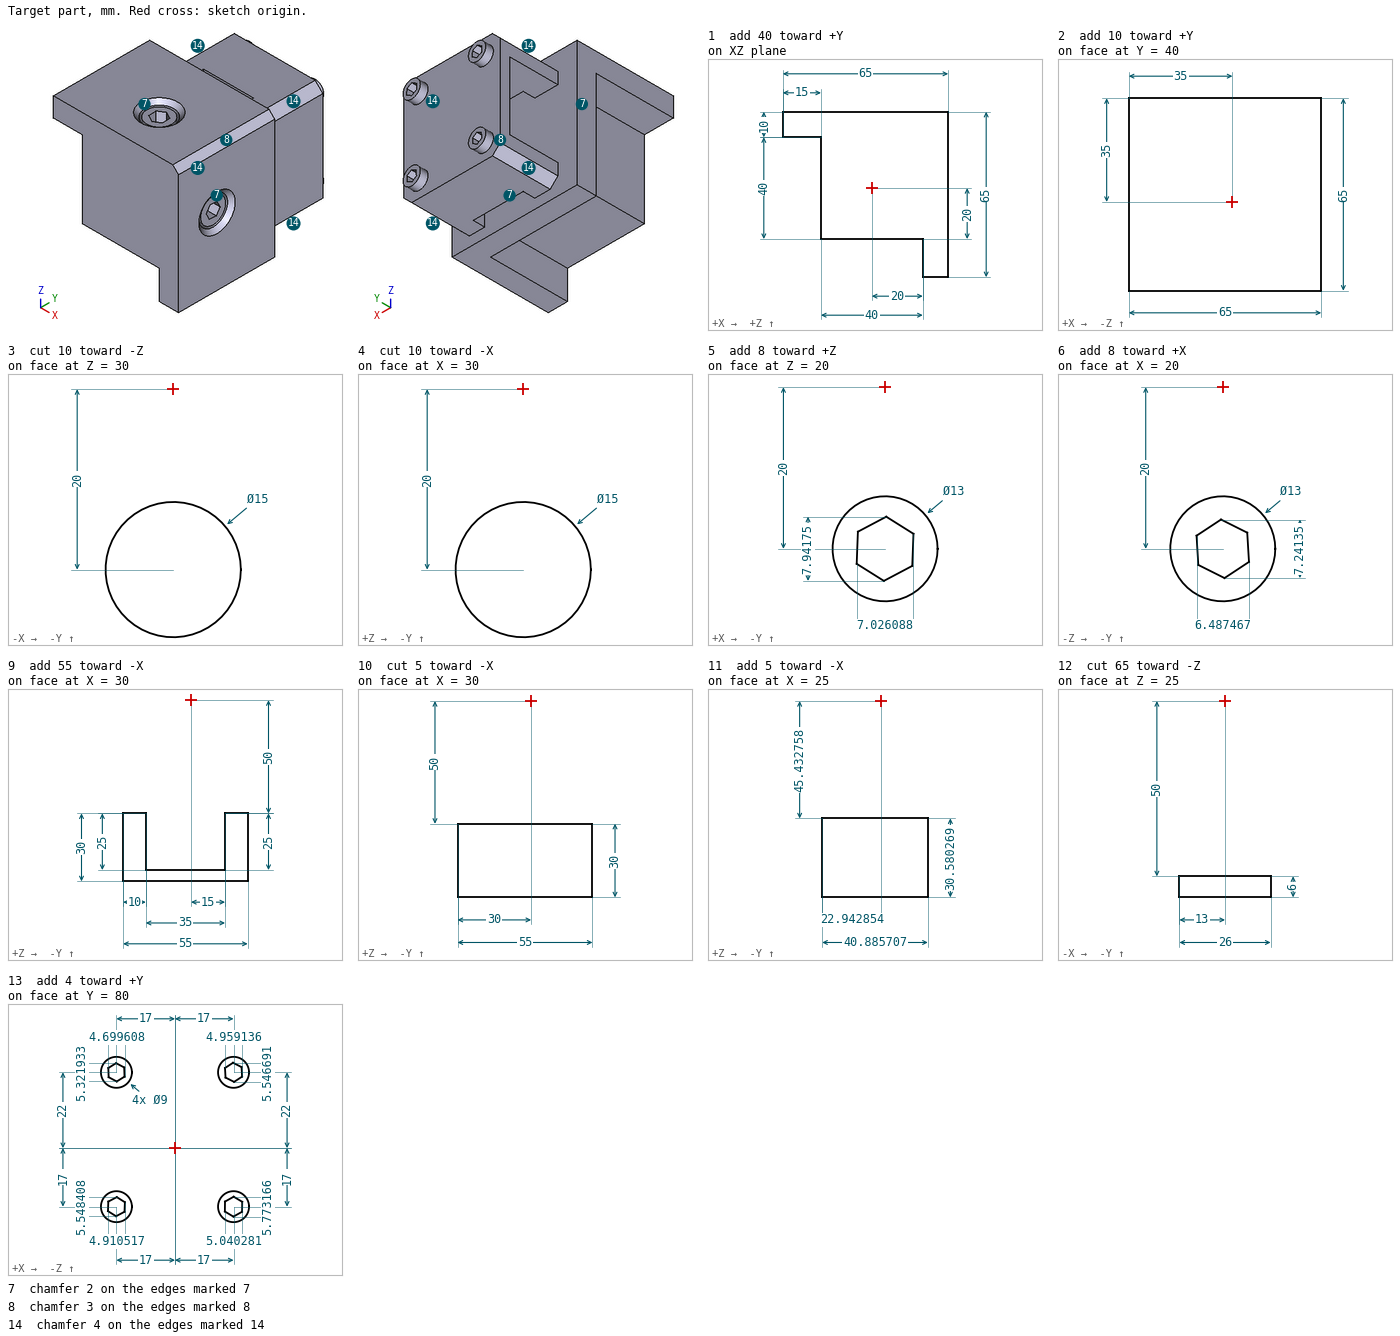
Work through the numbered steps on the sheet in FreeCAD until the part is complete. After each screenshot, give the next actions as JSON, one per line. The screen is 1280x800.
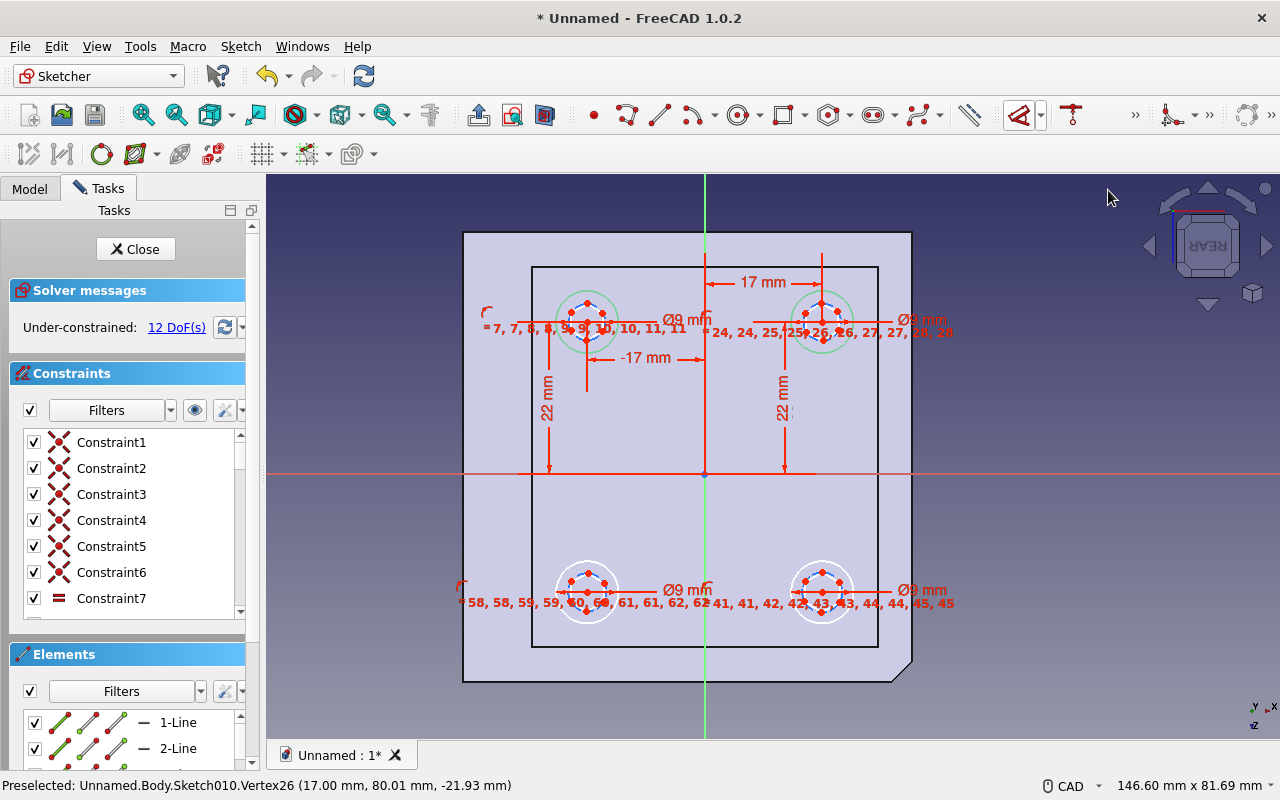
{"action": "left_click", "coordinate": [822, 592]}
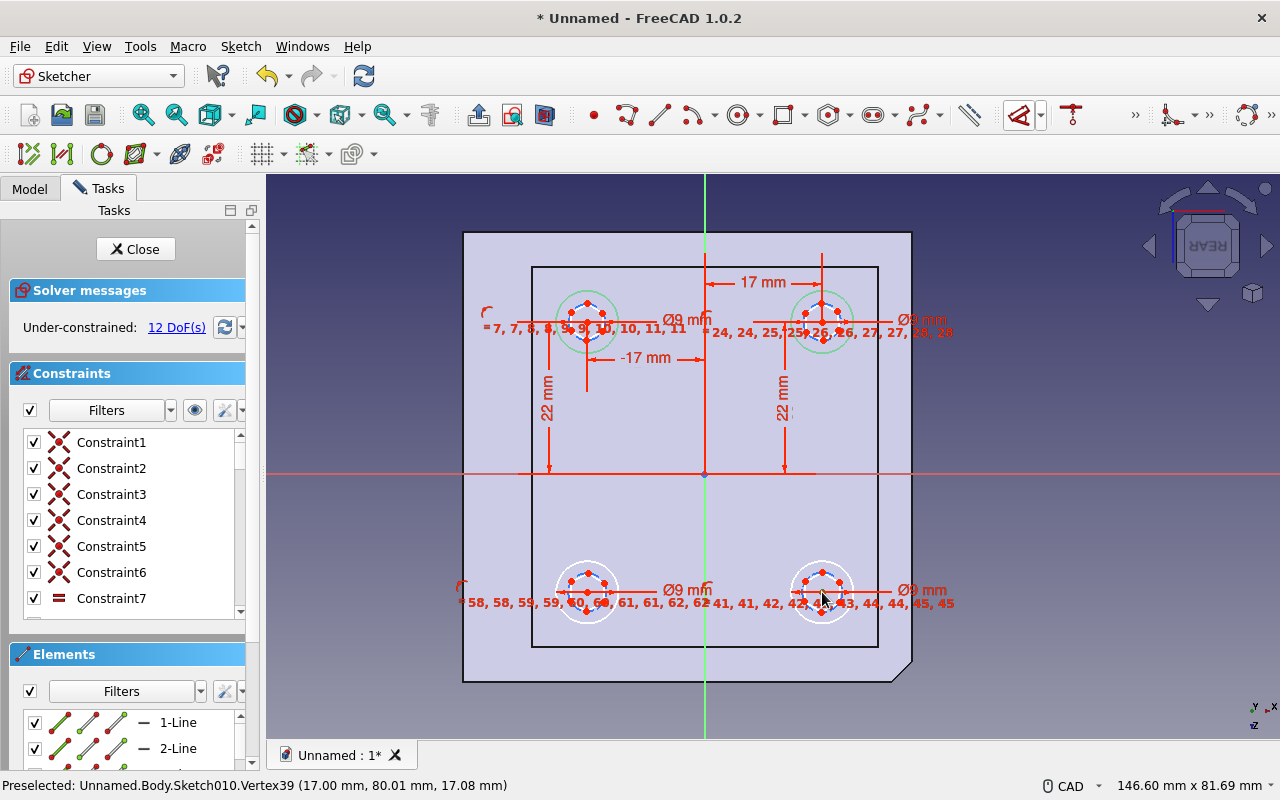
{"action": "left_click", "coordinate": [1040, 116]}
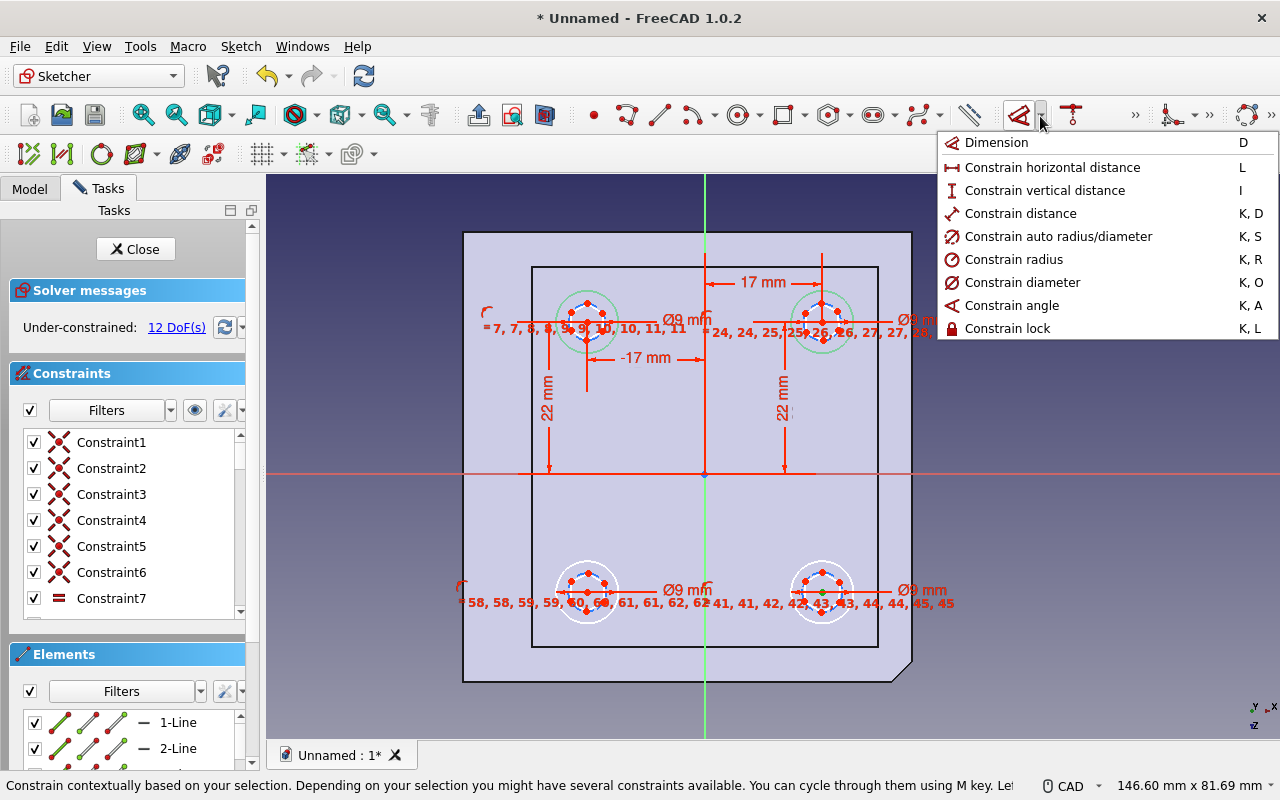
{"action": "left_click", "coordinate": [1108, 168]}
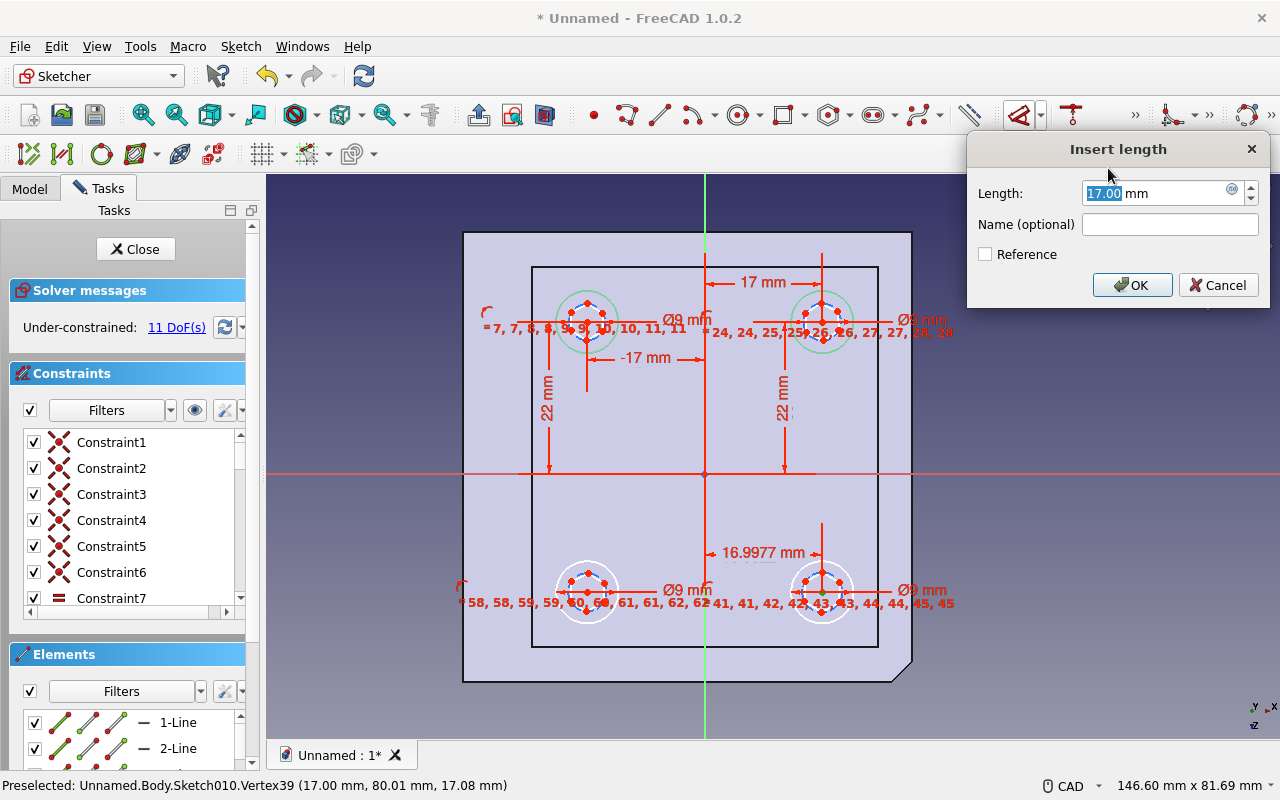
{"action": "type", "text": "17"}
{"action": "key", "text": "Return"}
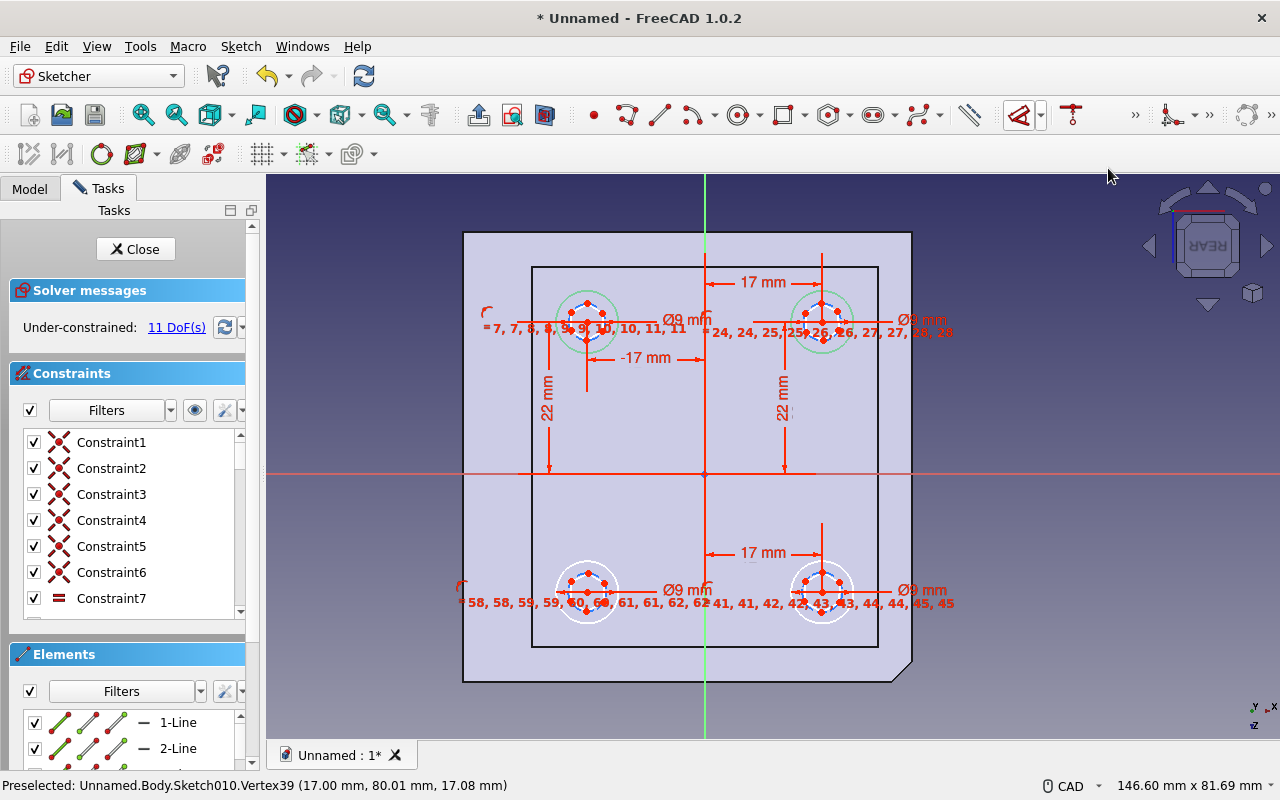
{"action": "left_click", "coordinate": [822, 592]}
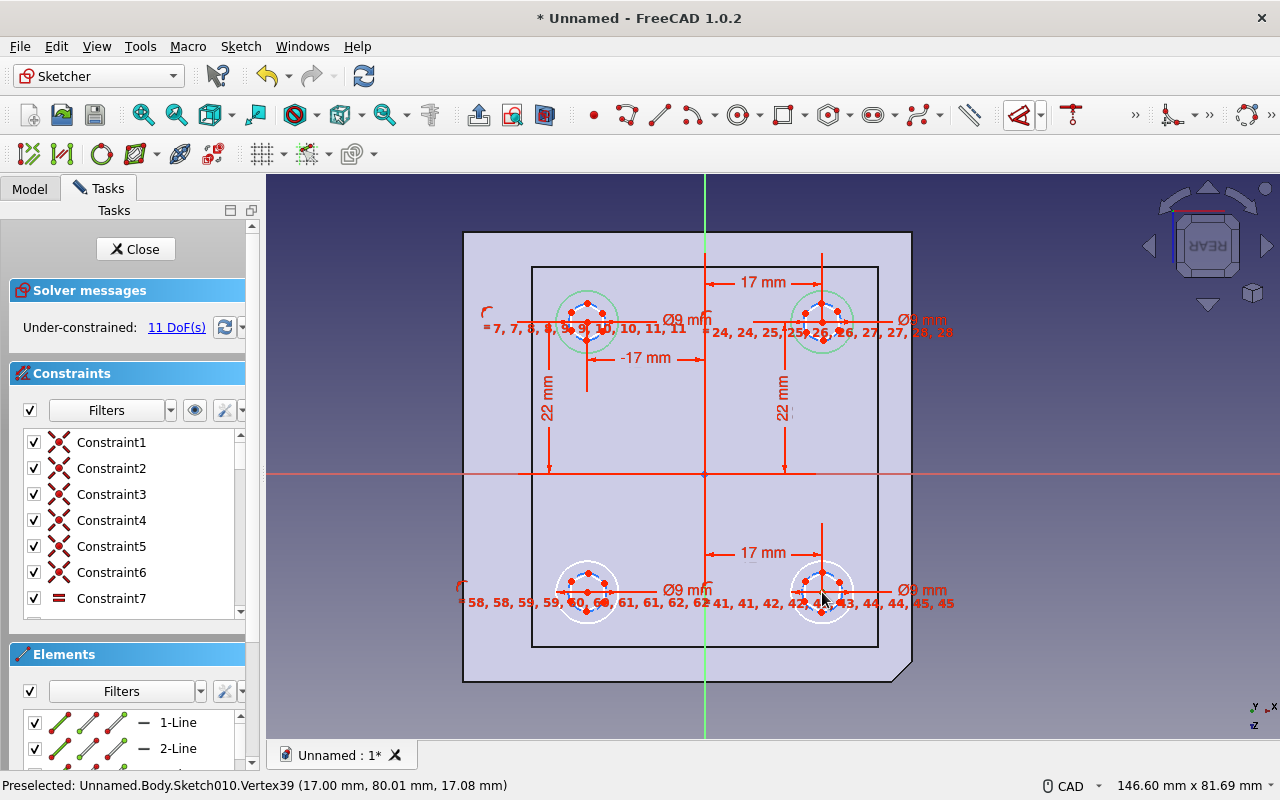
{"action": "key", "text": "i"}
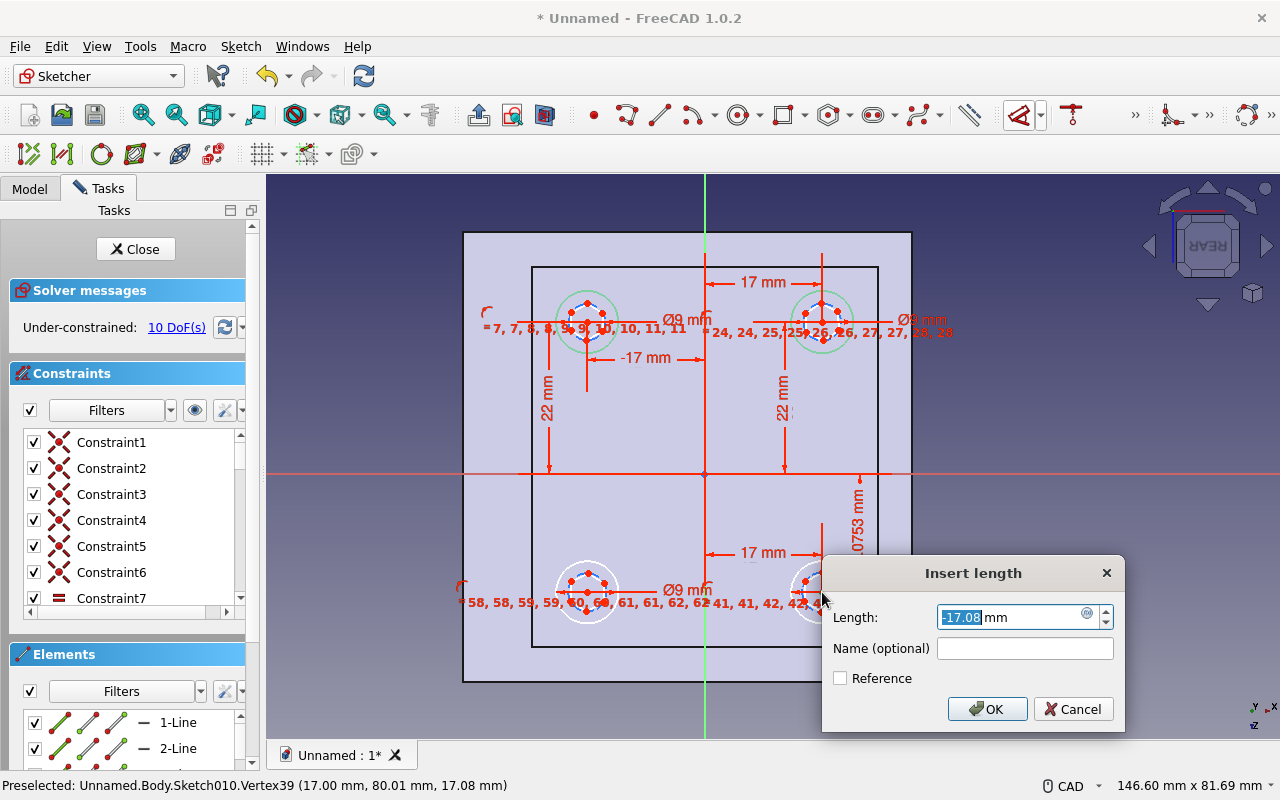
{"action": "type", "text": "-17"}
{"action": "key", "text": "Return"}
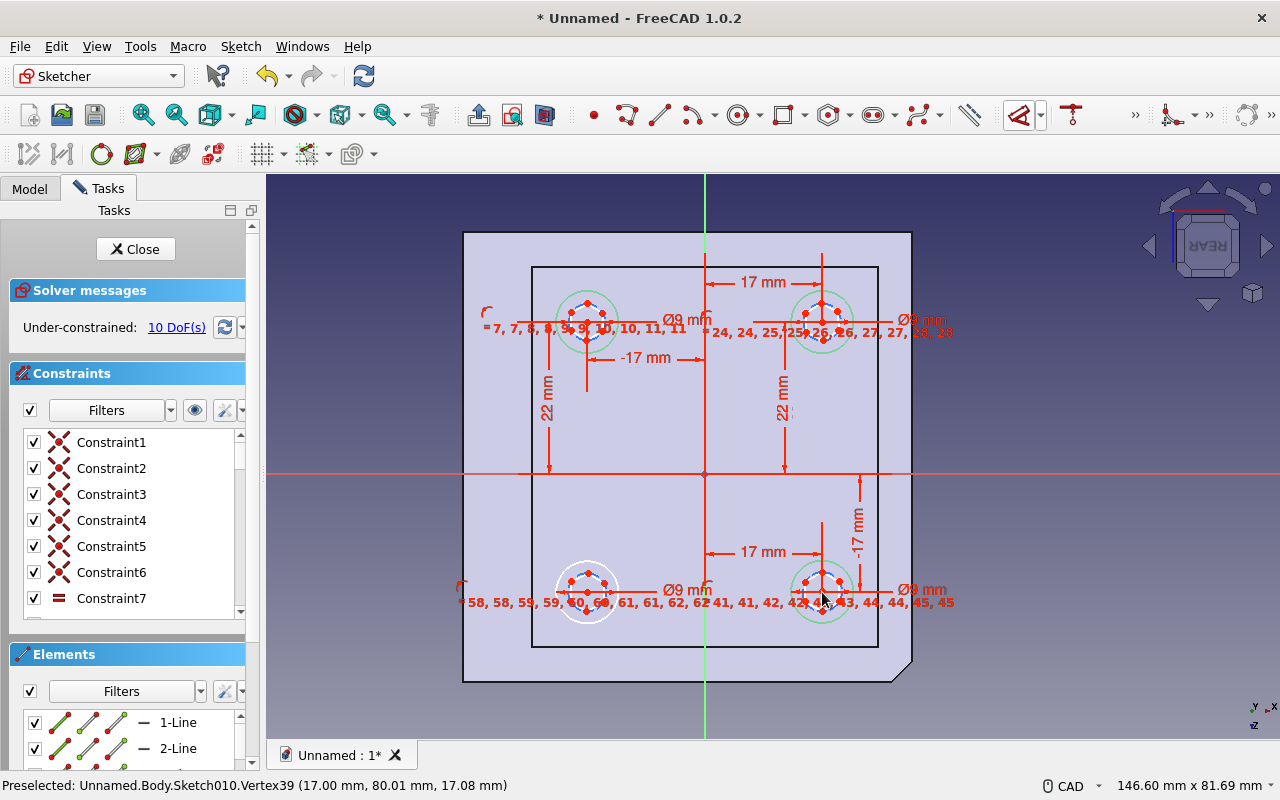
{"action": "left_click", "coordinate": [587, 592]}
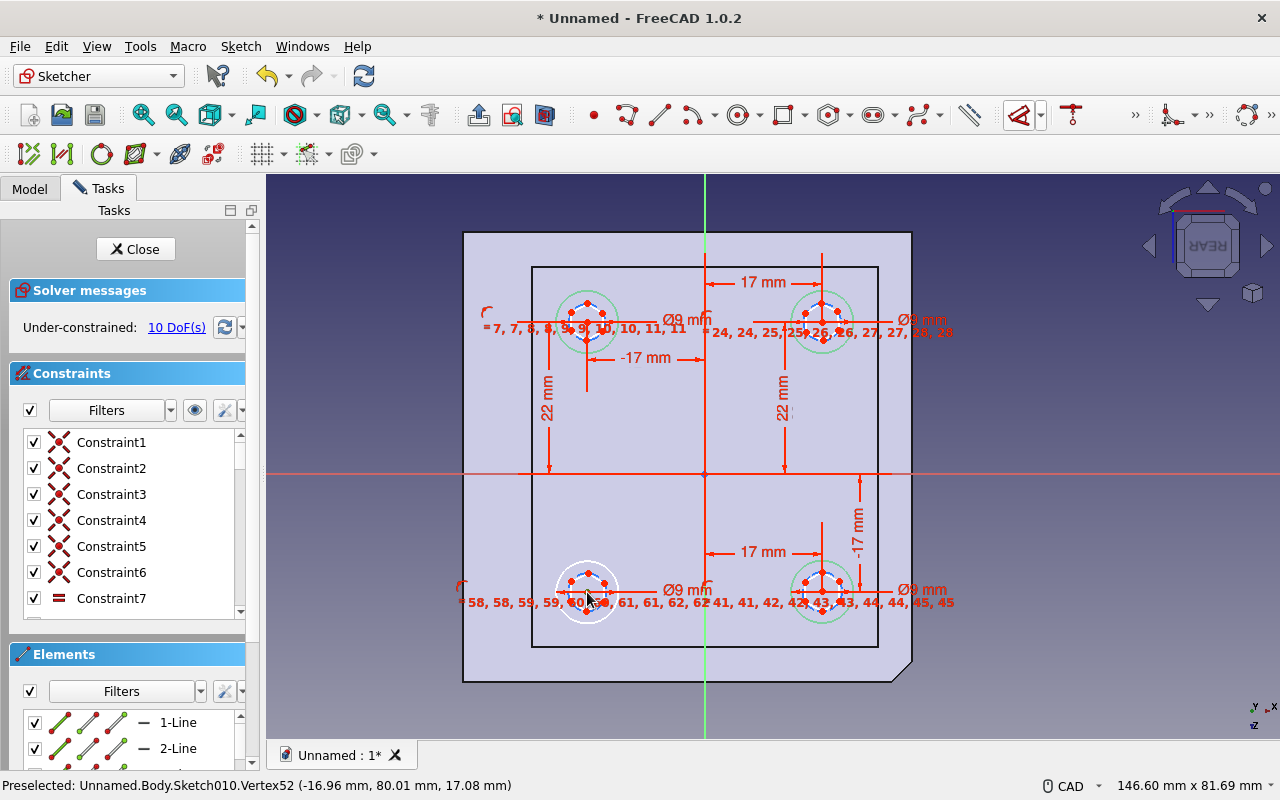
{"action": "left_click", "coordinate": [1040, 116]}